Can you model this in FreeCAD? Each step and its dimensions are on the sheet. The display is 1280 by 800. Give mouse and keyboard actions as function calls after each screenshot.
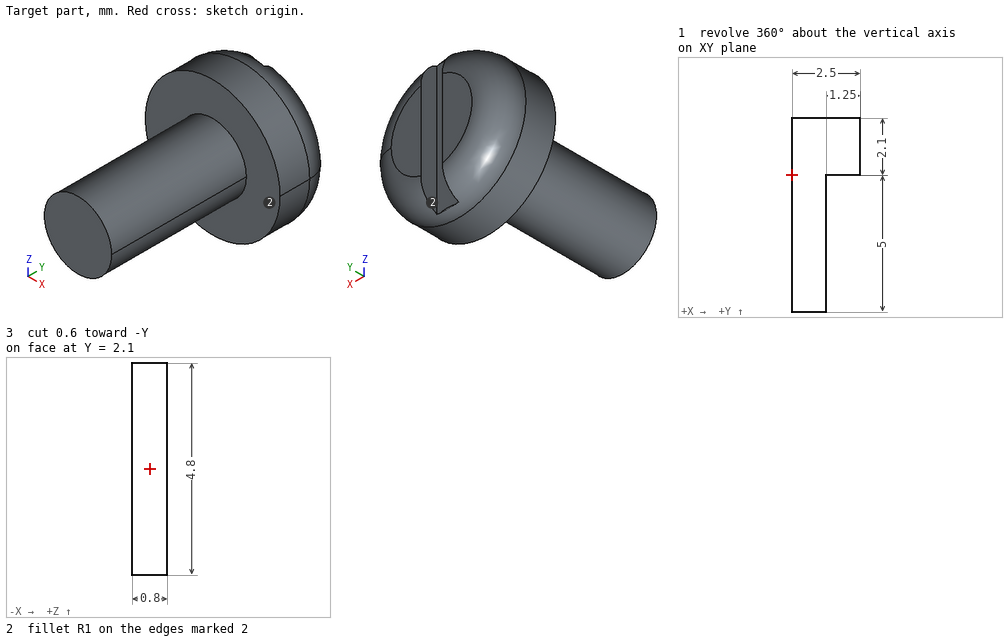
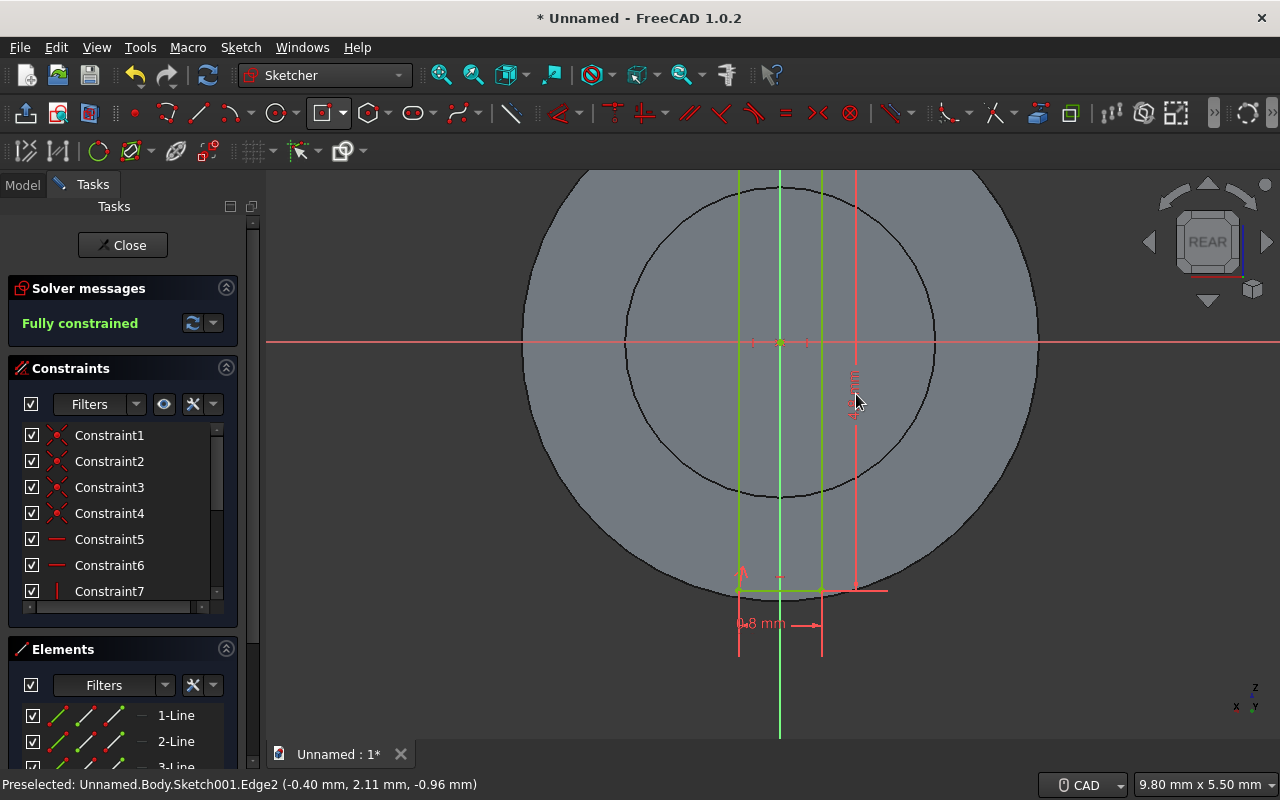
click(123, 245)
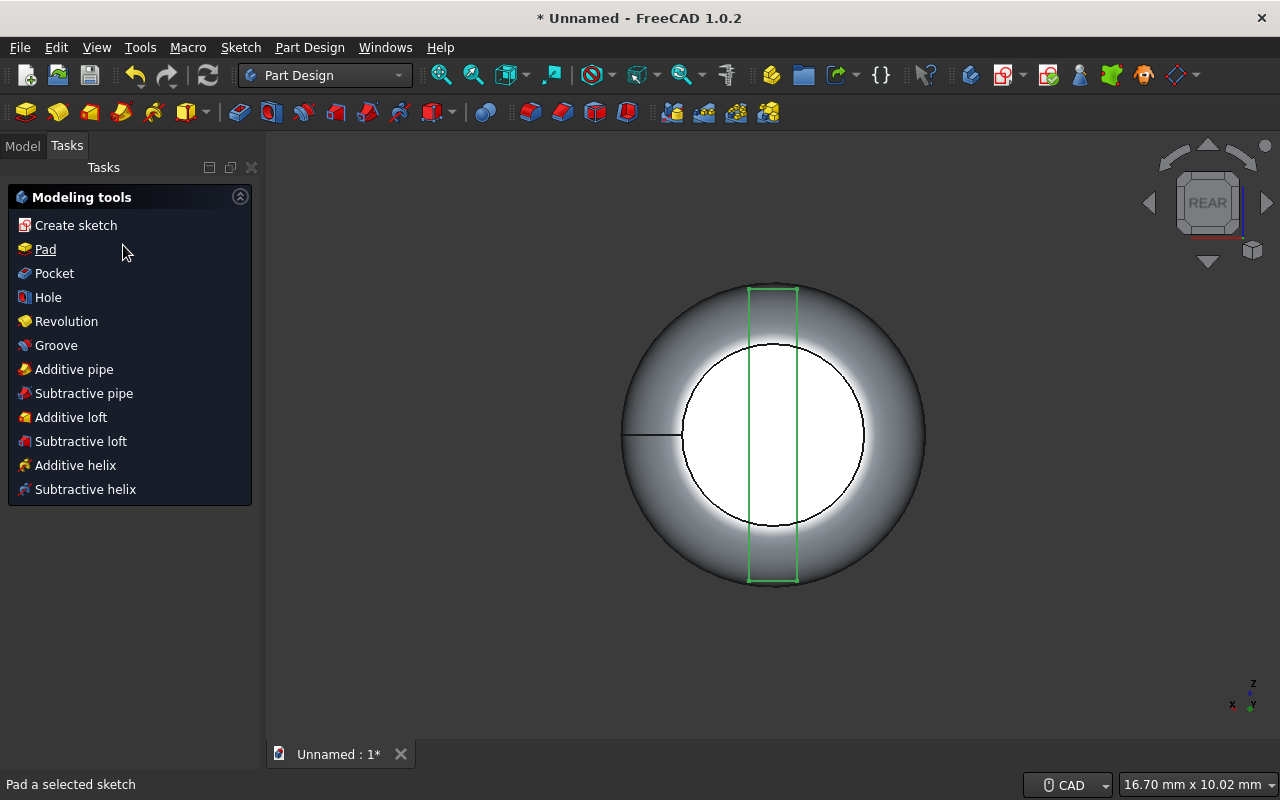
click(240, 112)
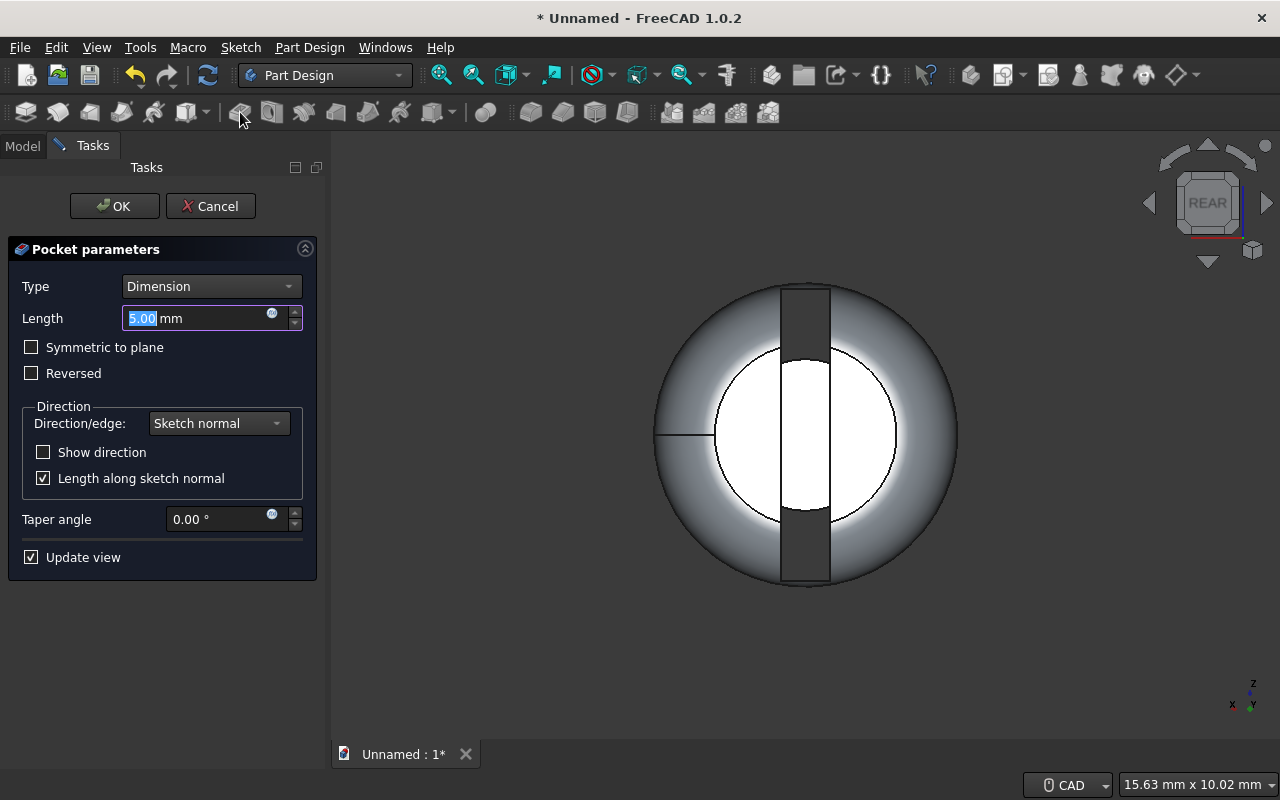
text(0.6)
key(Tab)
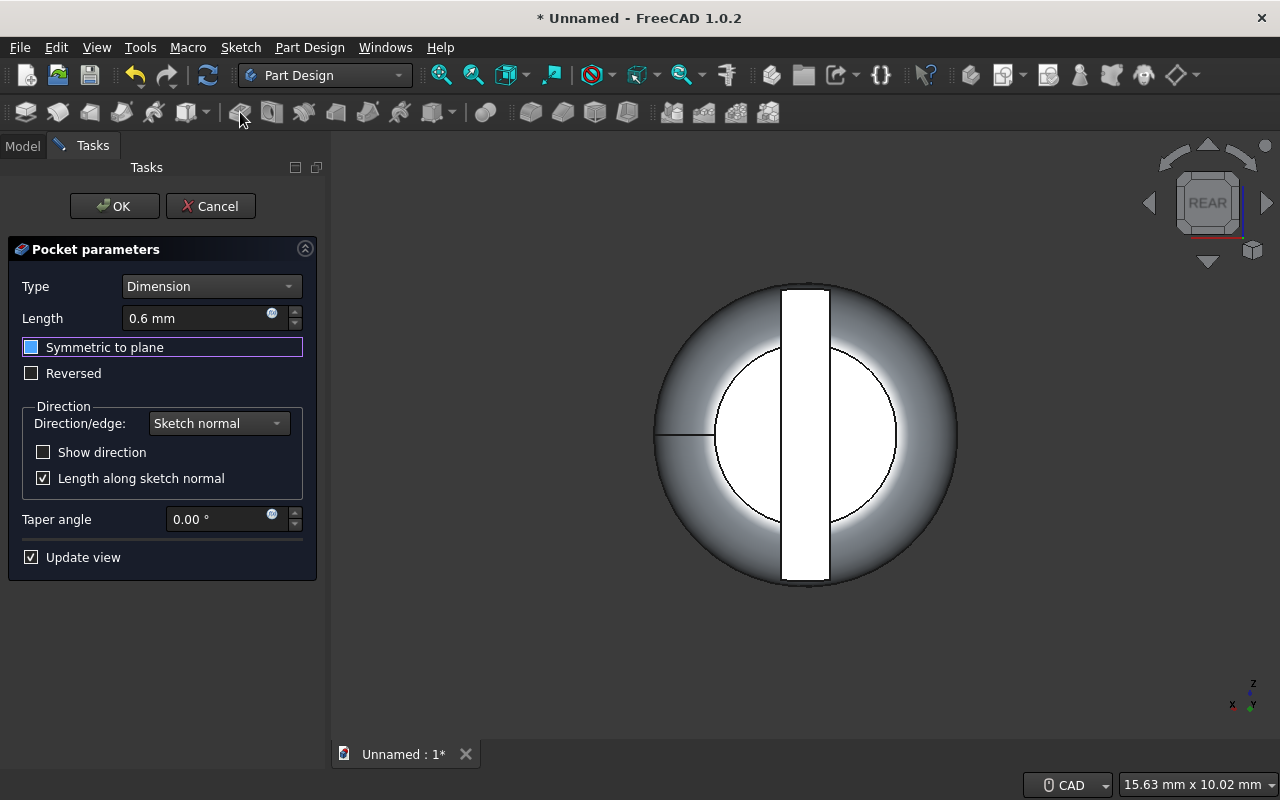
click(115, 206)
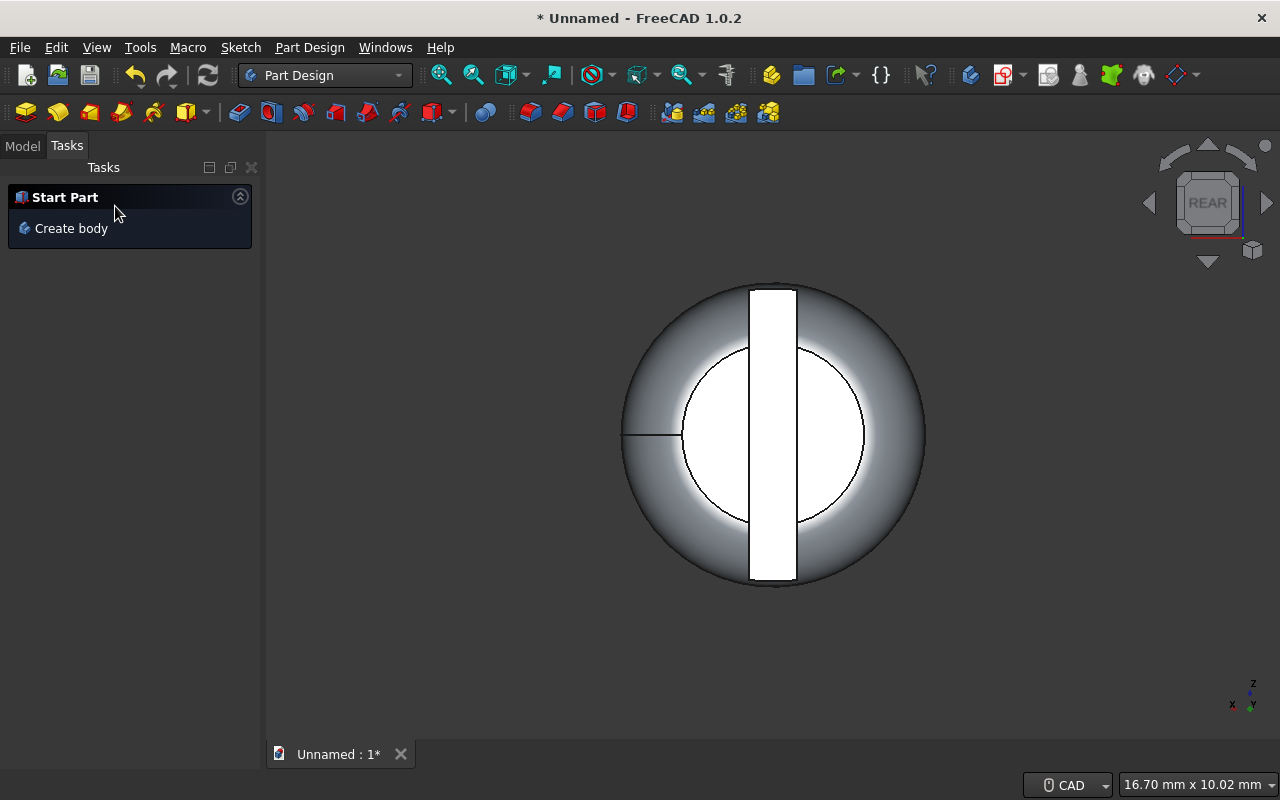
key(0)